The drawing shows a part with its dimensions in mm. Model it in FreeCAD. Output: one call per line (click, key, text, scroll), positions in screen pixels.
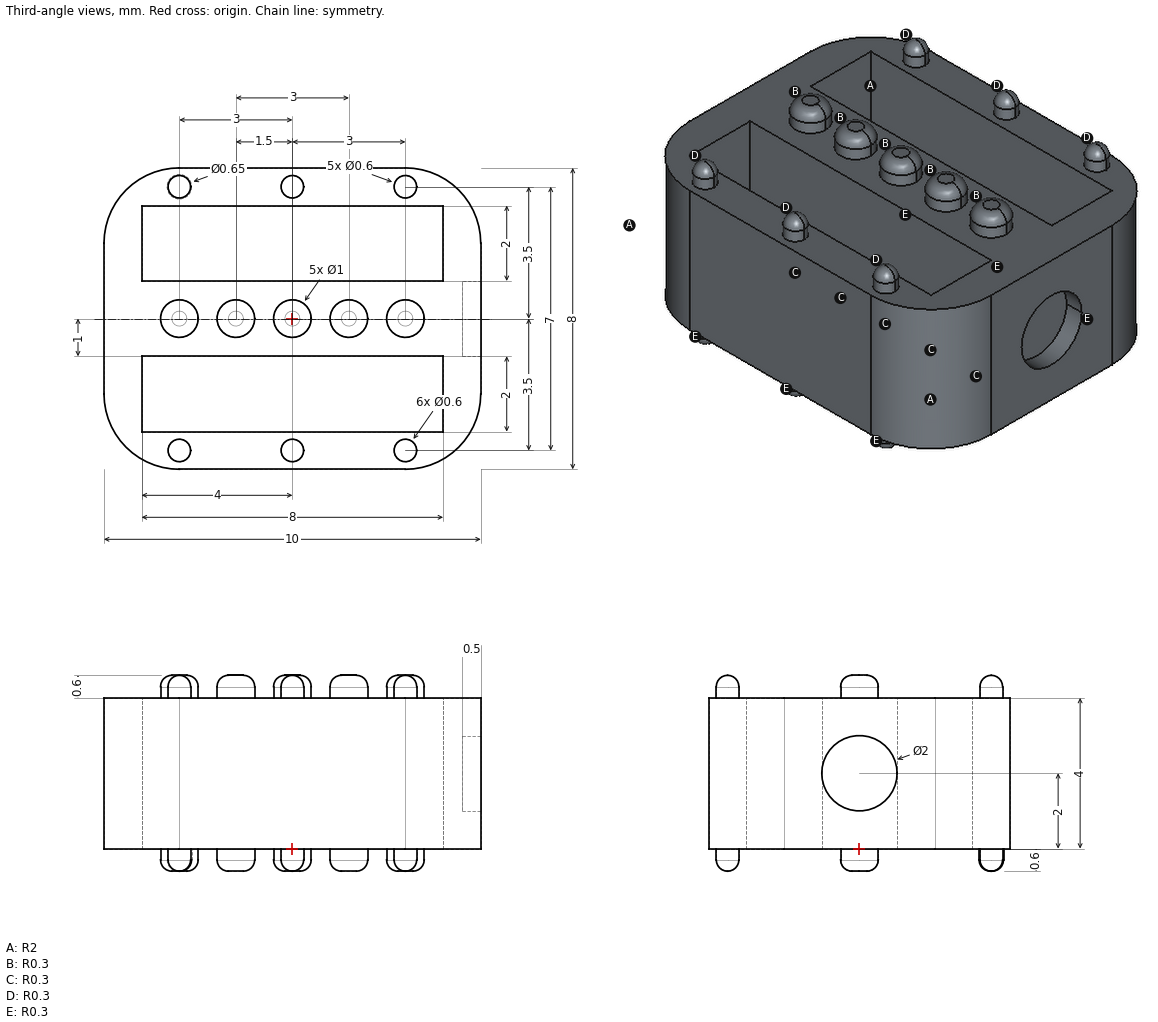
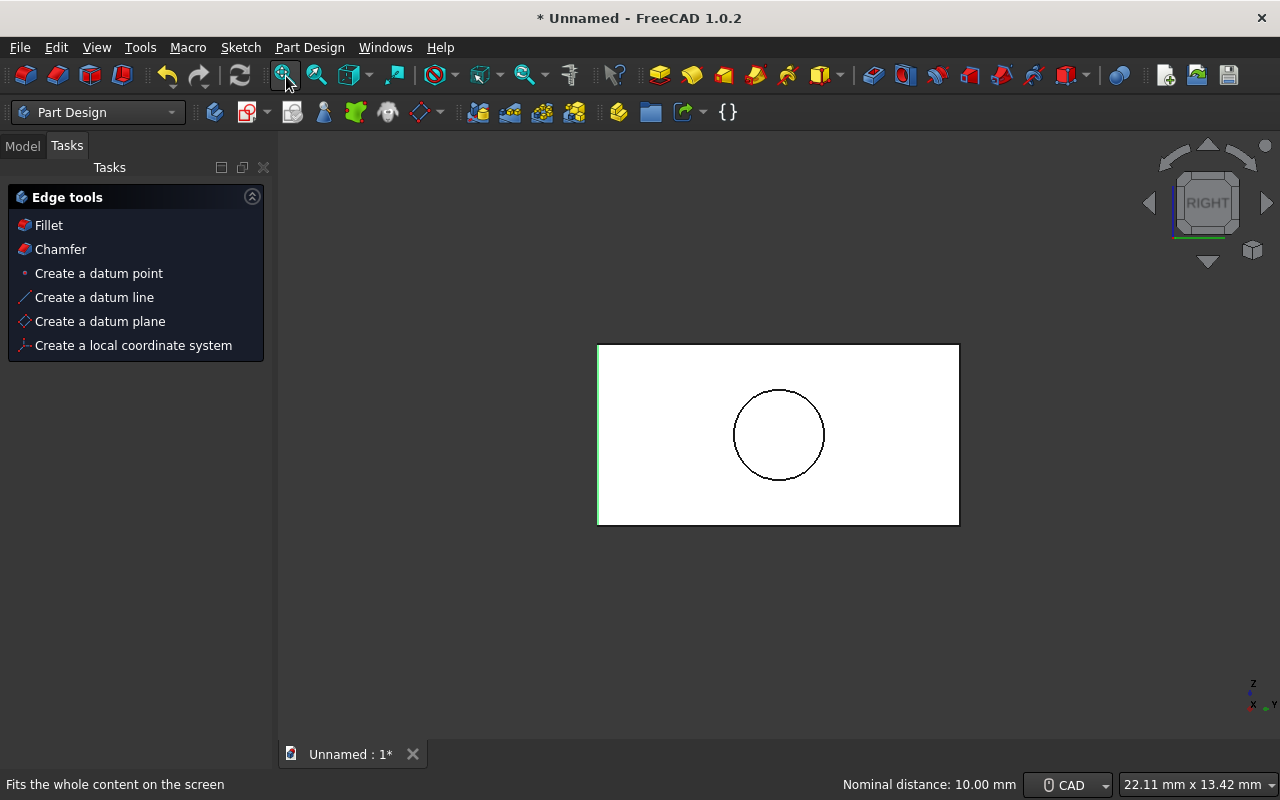
click(960, 434, ctrl)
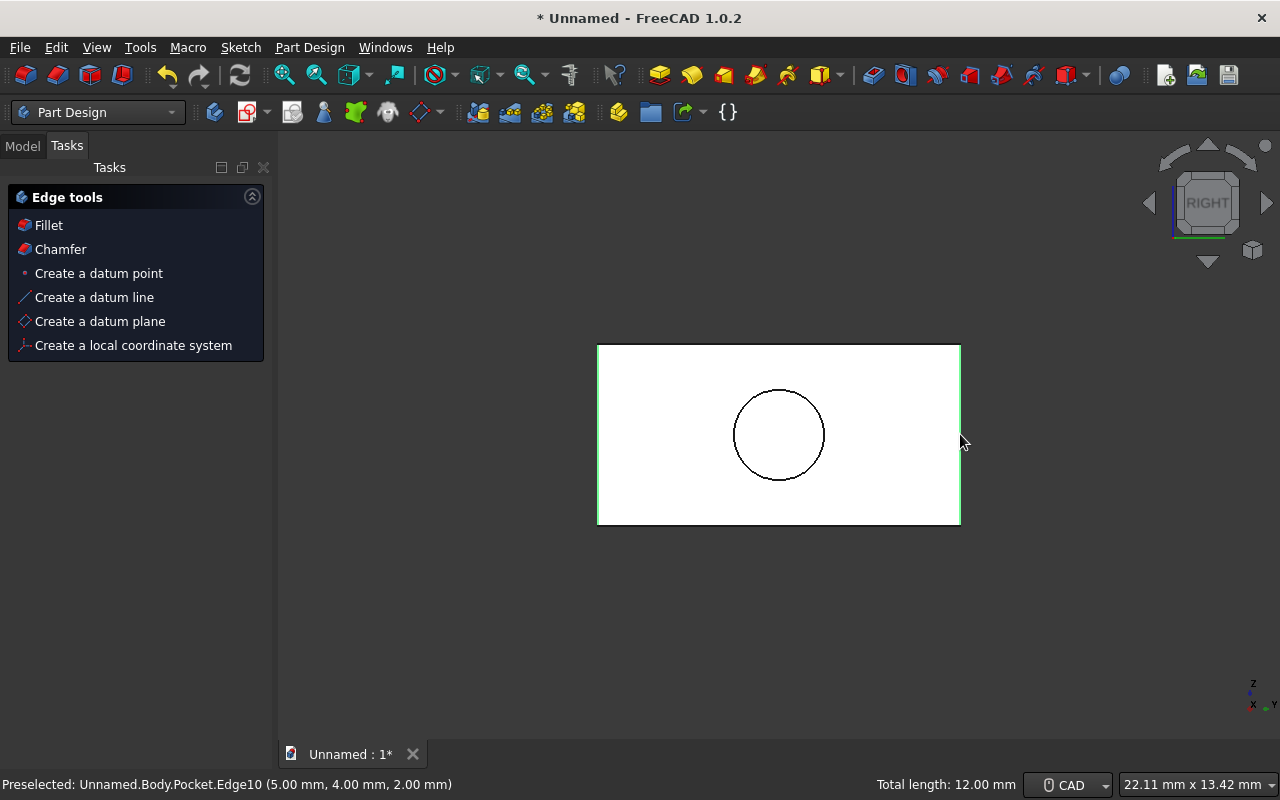
key(5)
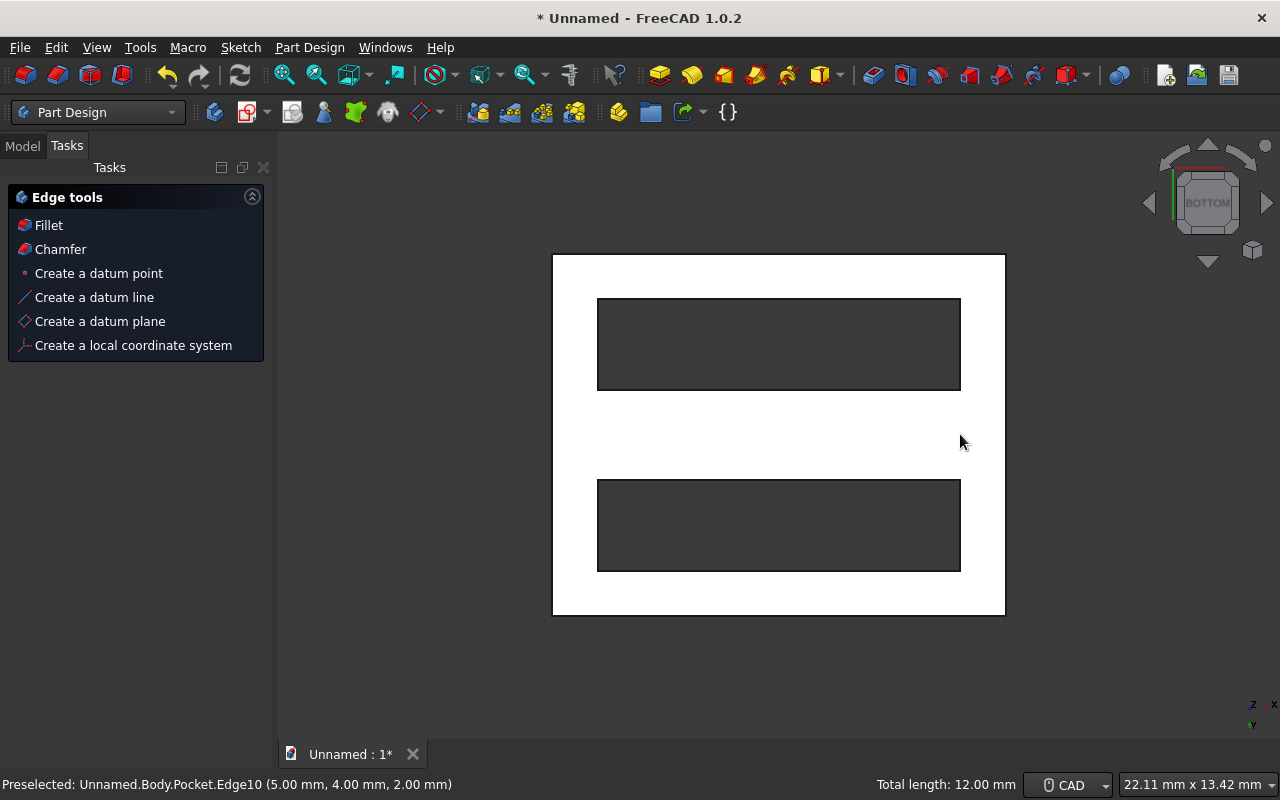
key(4)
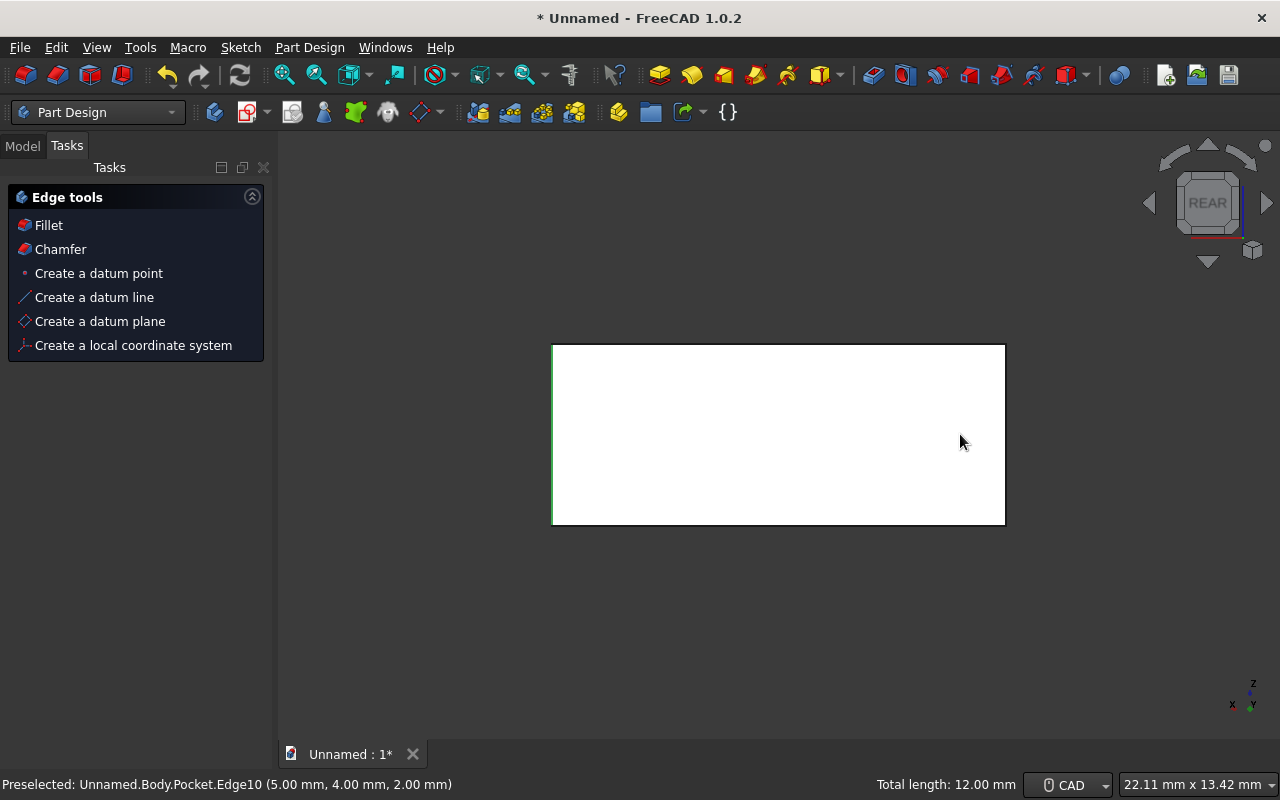
click(1006, 434, ctrl)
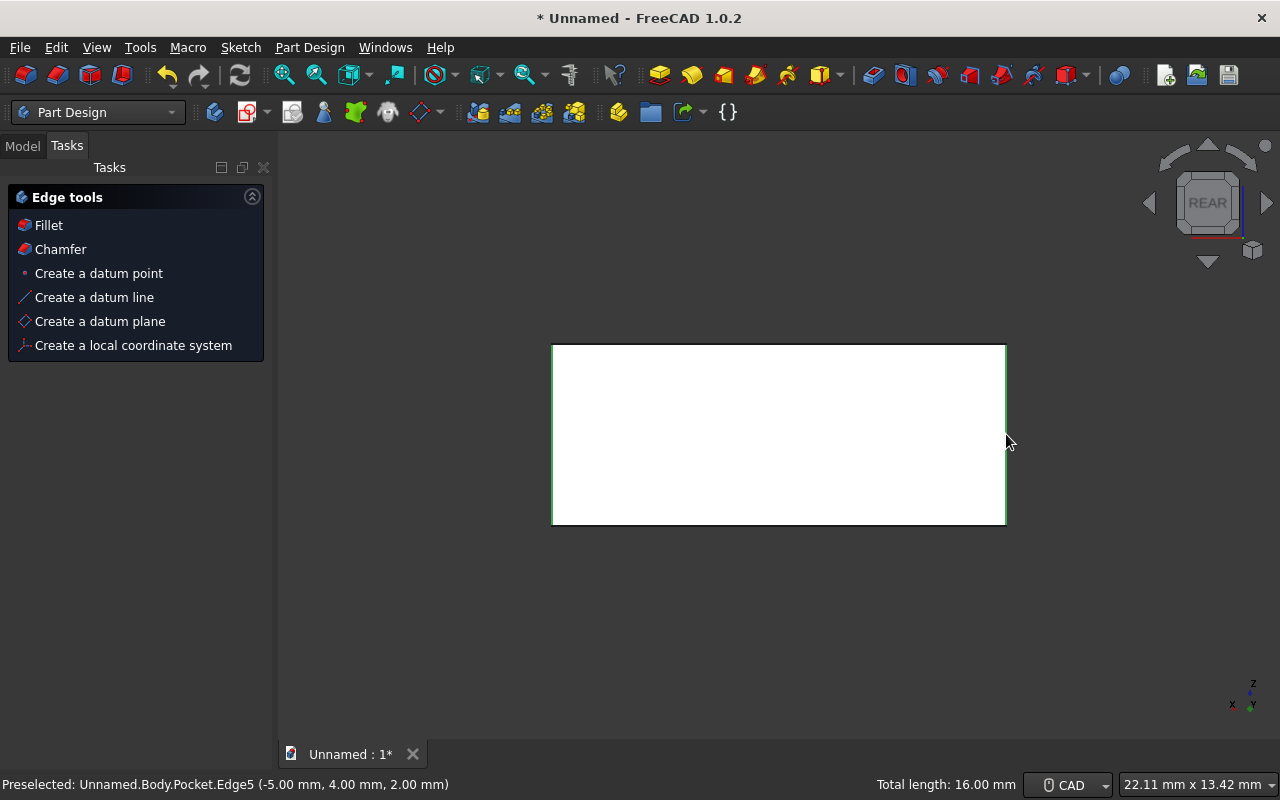
click(26, 76)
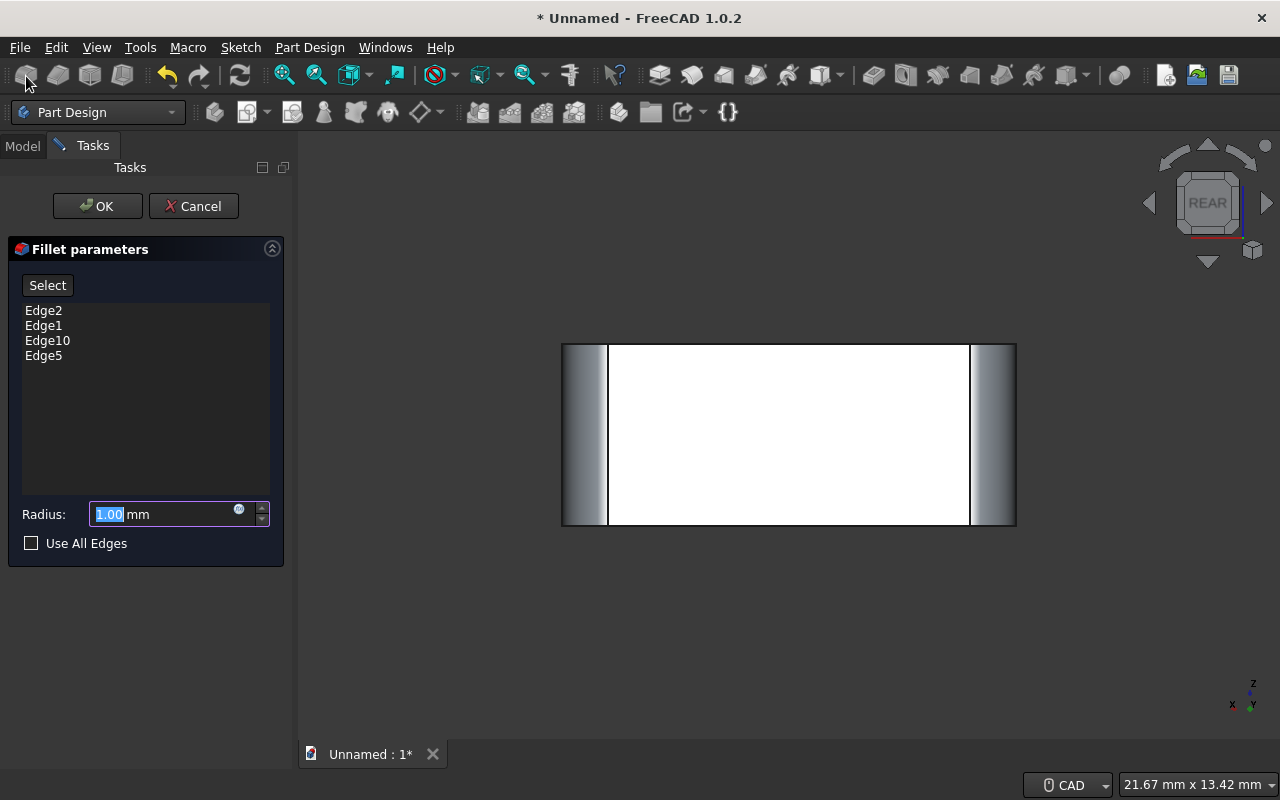
text(2)
key(Tab)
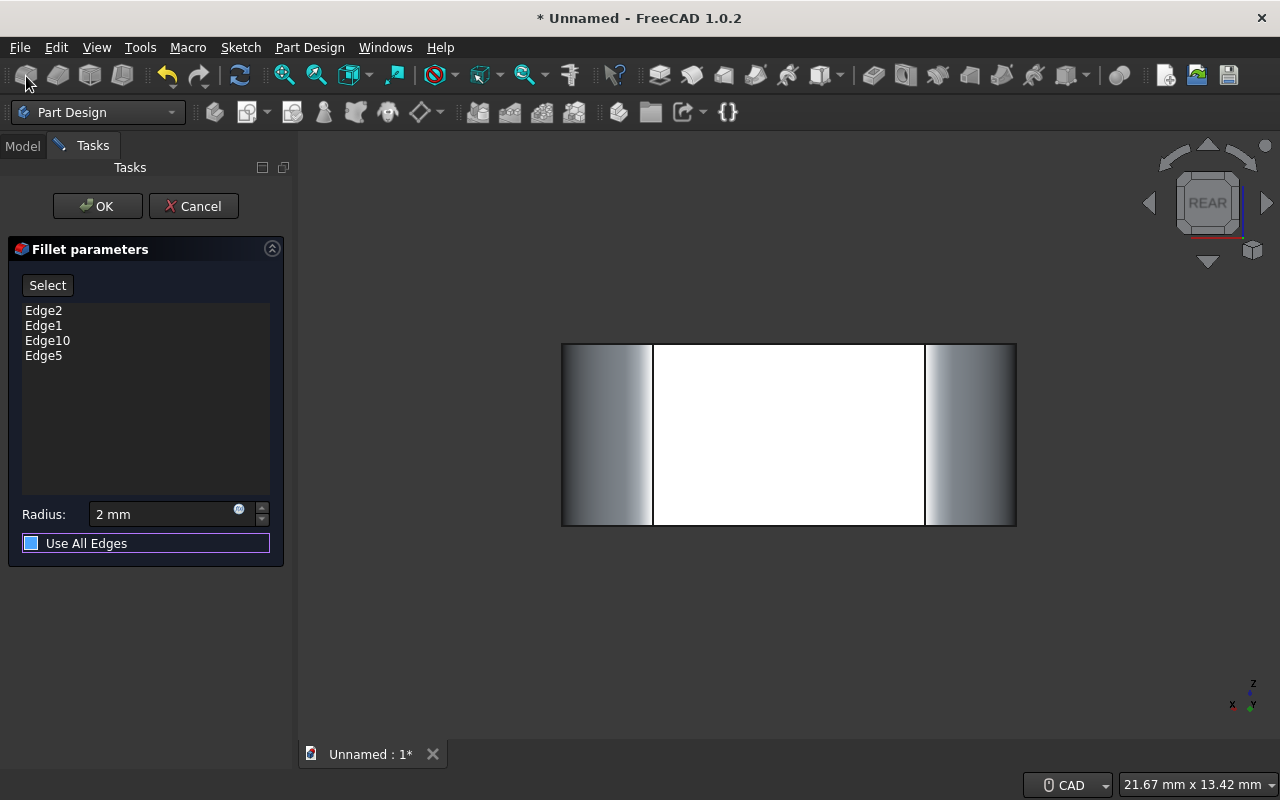
click(98, 206)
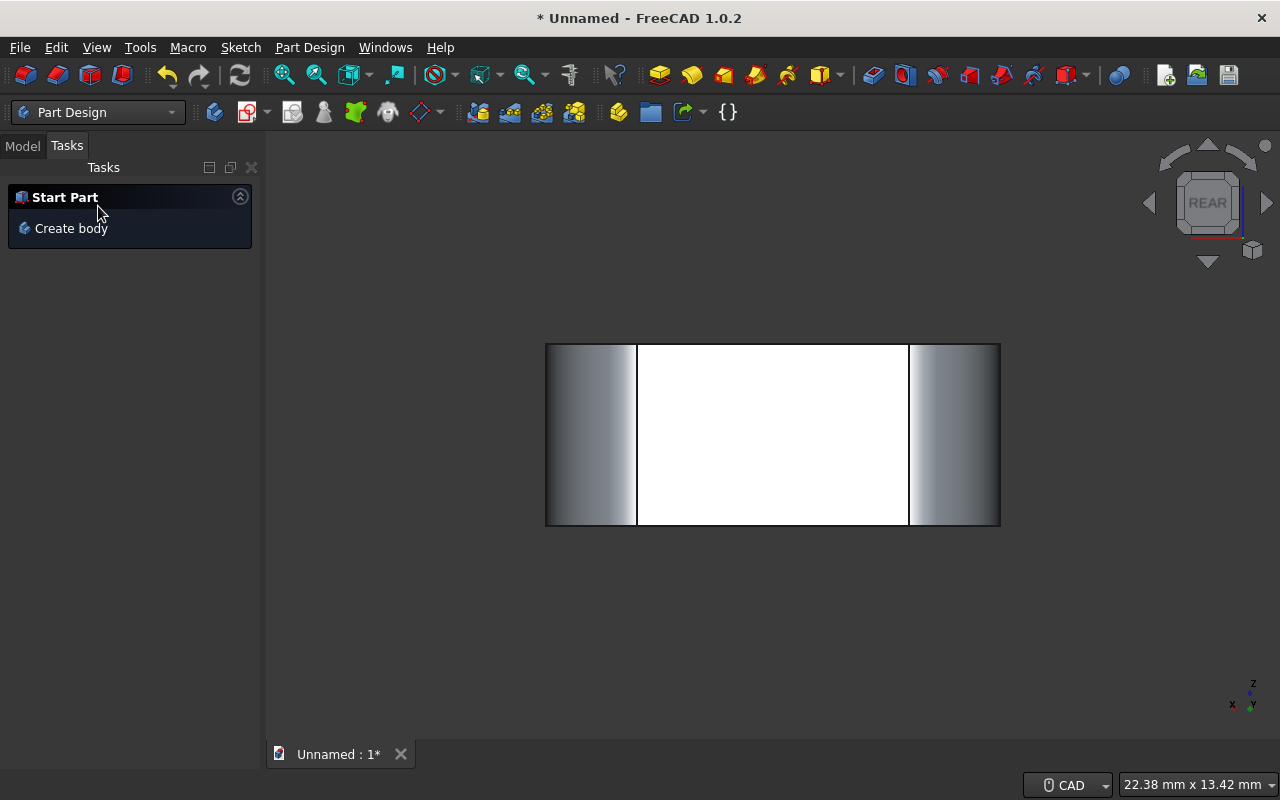
click(286, 76)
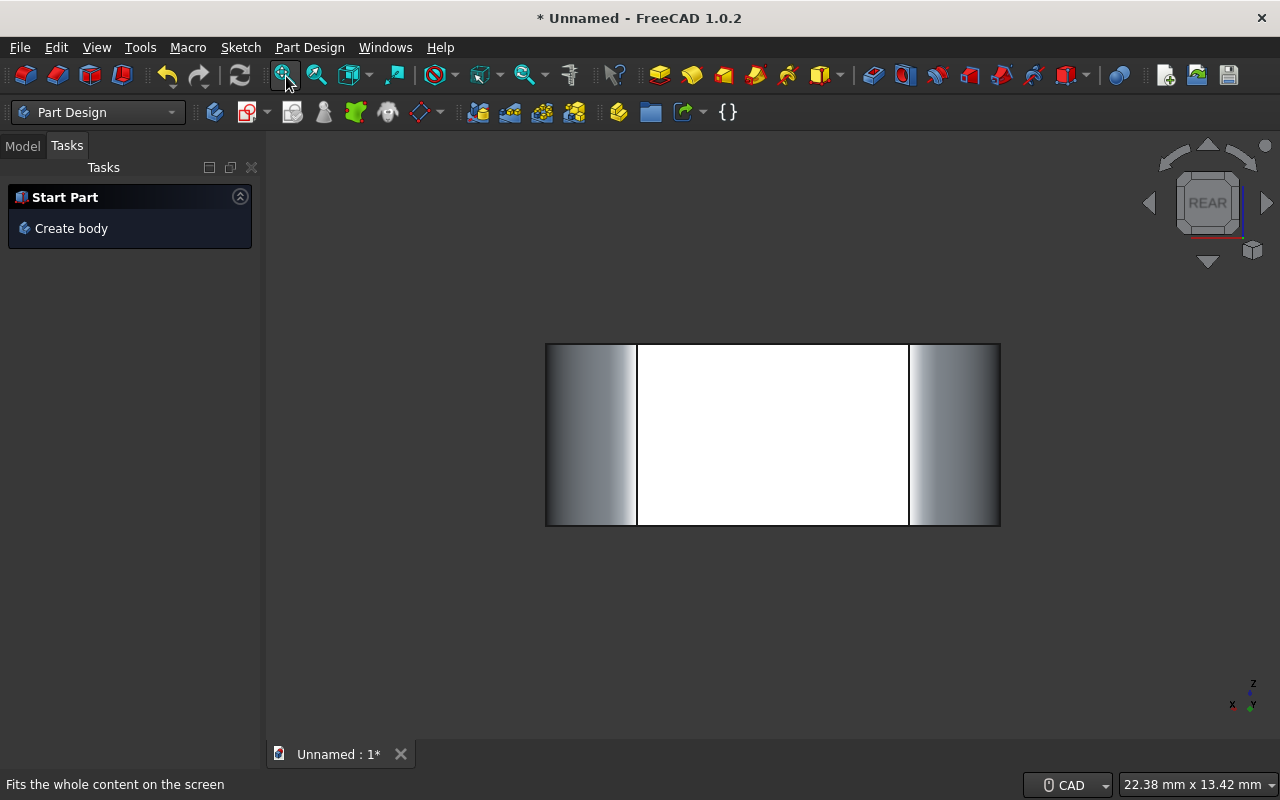
key(0)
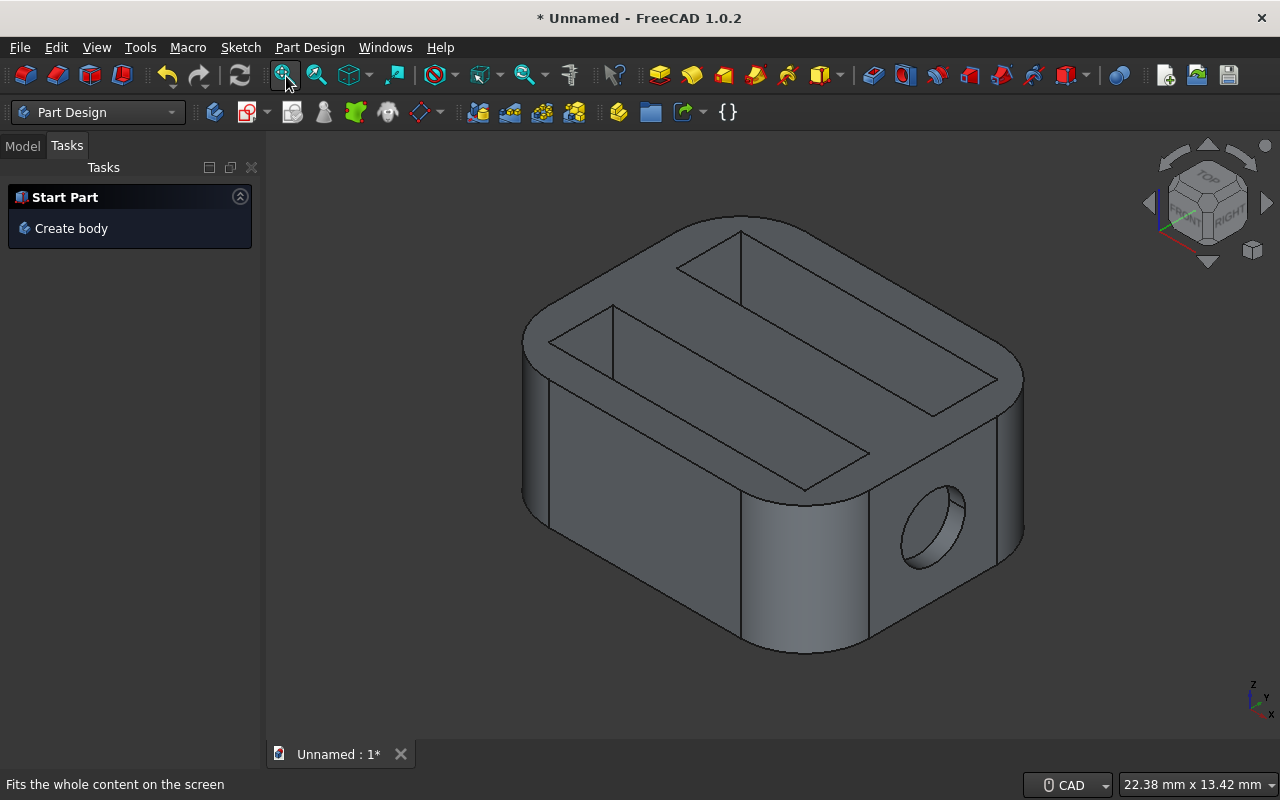
click(865, 413)